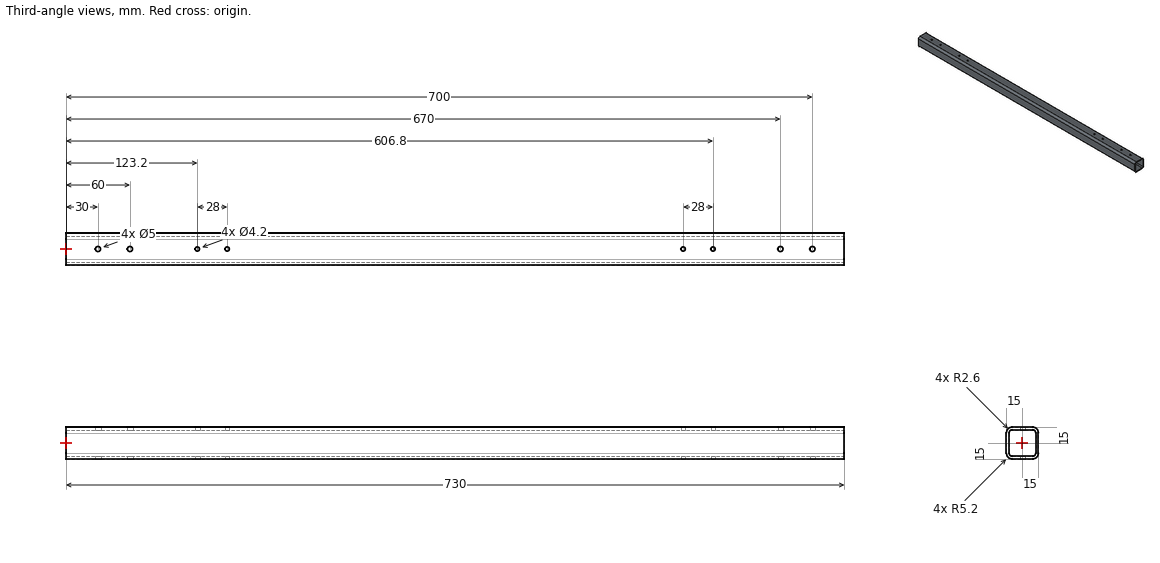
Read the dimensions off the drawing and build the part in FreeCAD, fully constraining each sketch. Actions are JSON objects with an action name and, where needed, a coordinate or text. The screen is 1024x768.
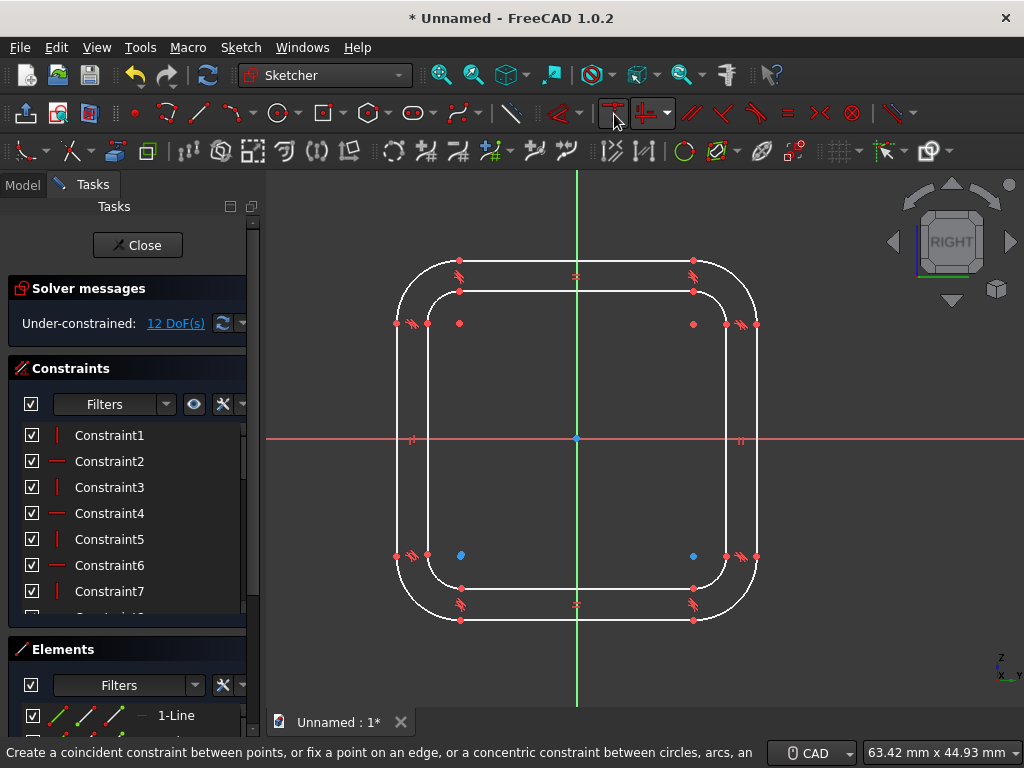
{"action": "left_click", "coordinate": [722, 613]}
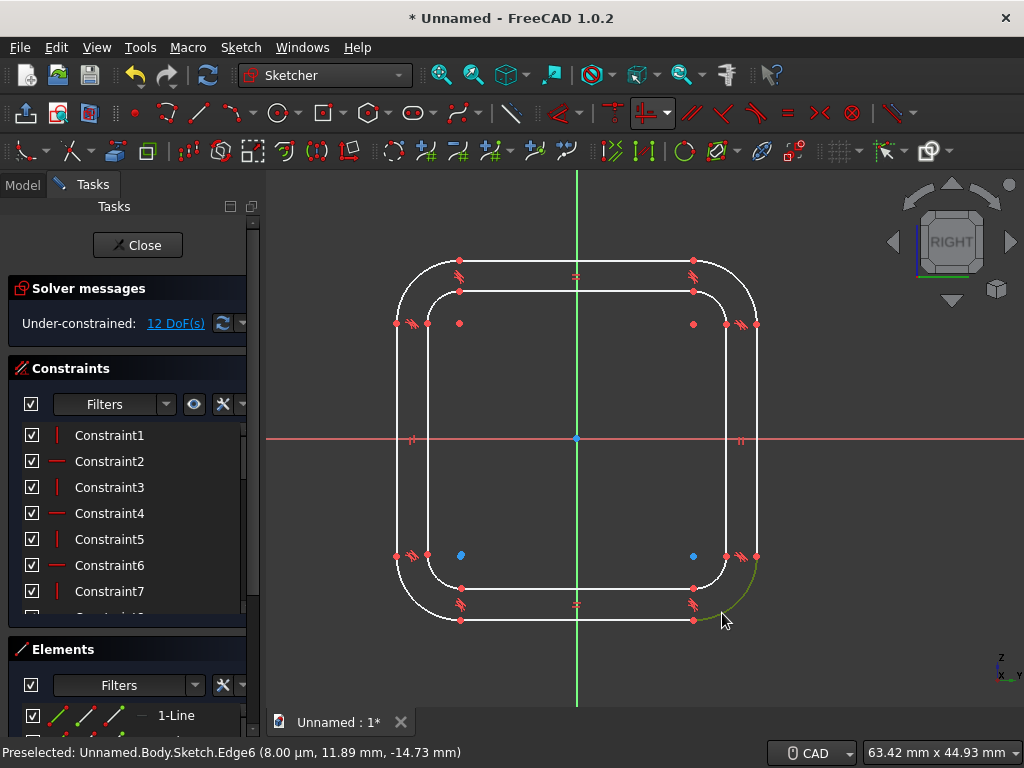
{"action": "left_click", "coordinate": [709, 585]}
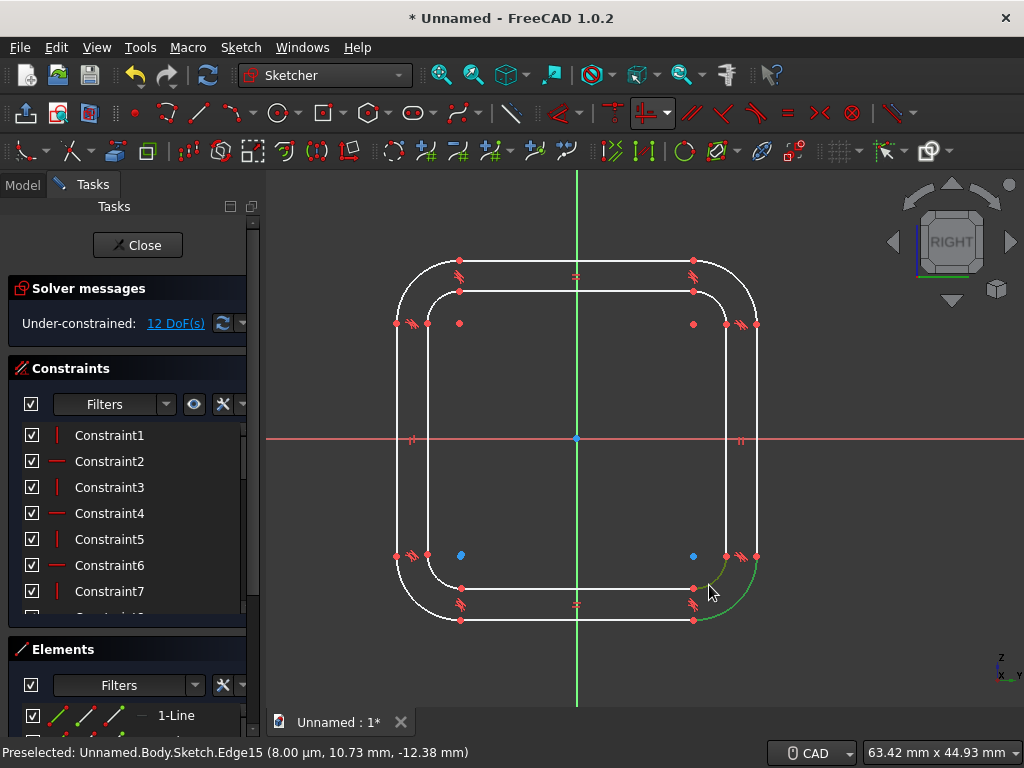
{"action": "left_click", "coordinate": [614, 114]}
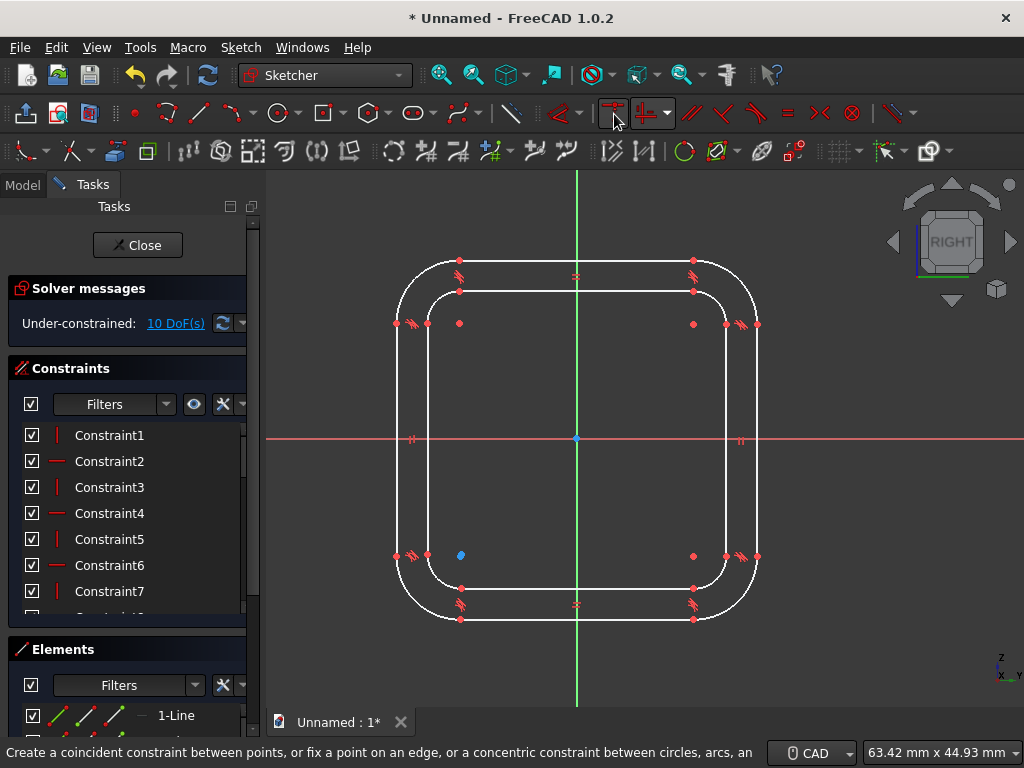
{"action": "left_click", "coordinate": [404, 585]}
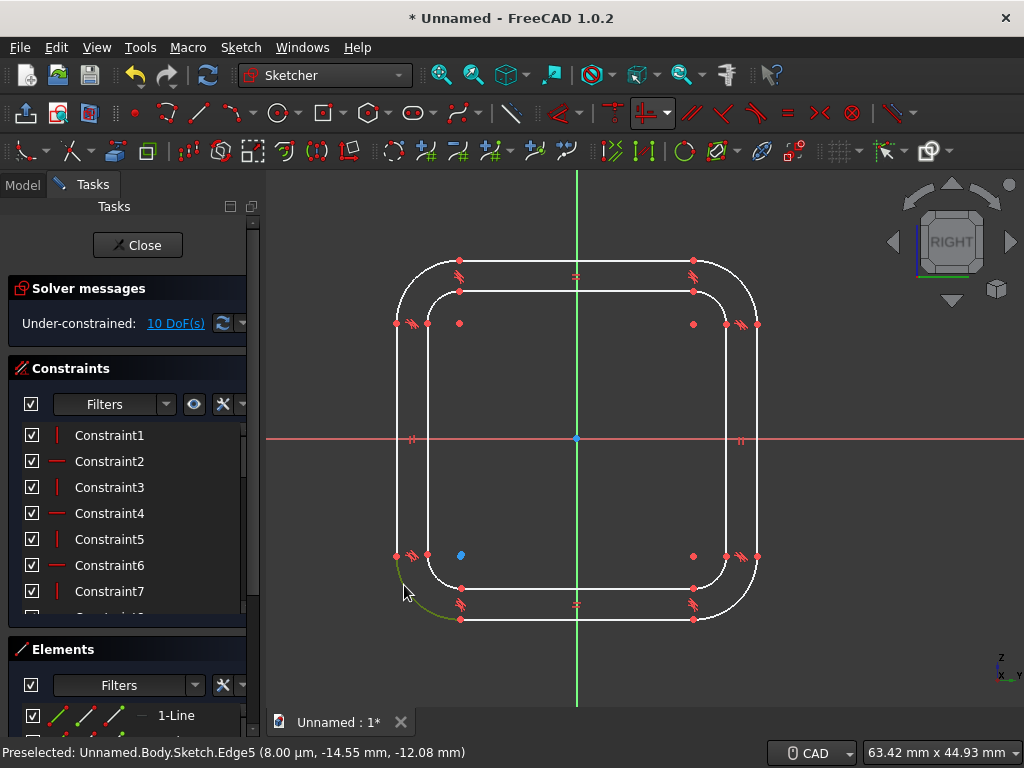
{"action": "left_click", "coordinate": [723, 613]}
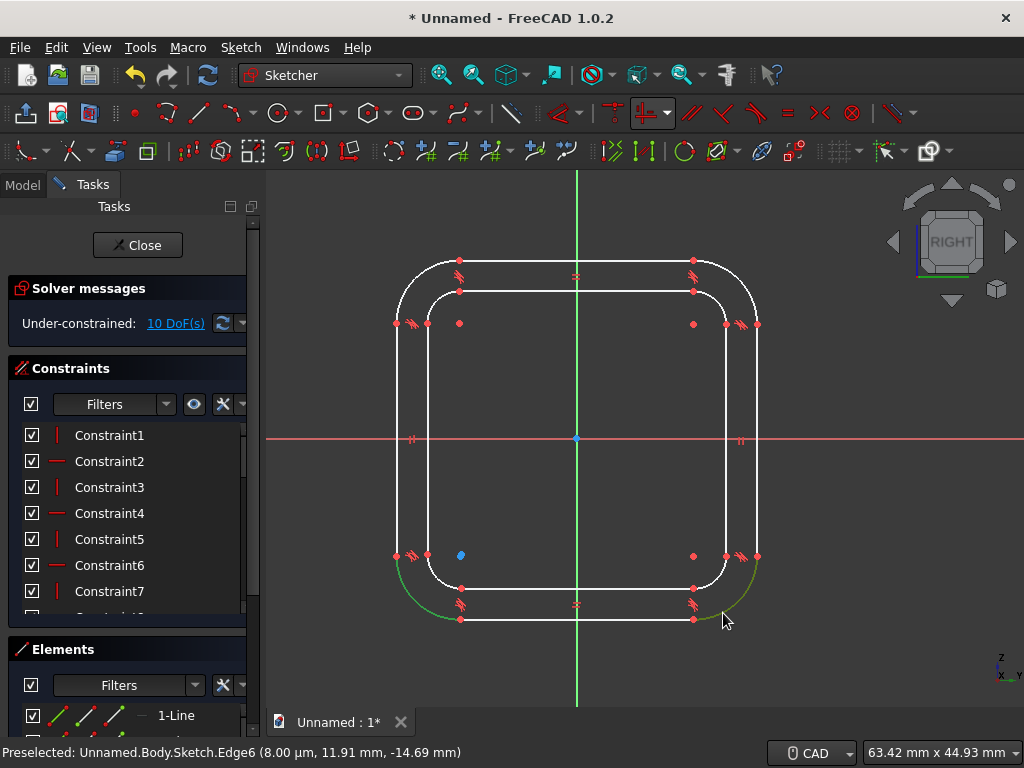
{"action": "left_click", "coordinate": [750, 295]}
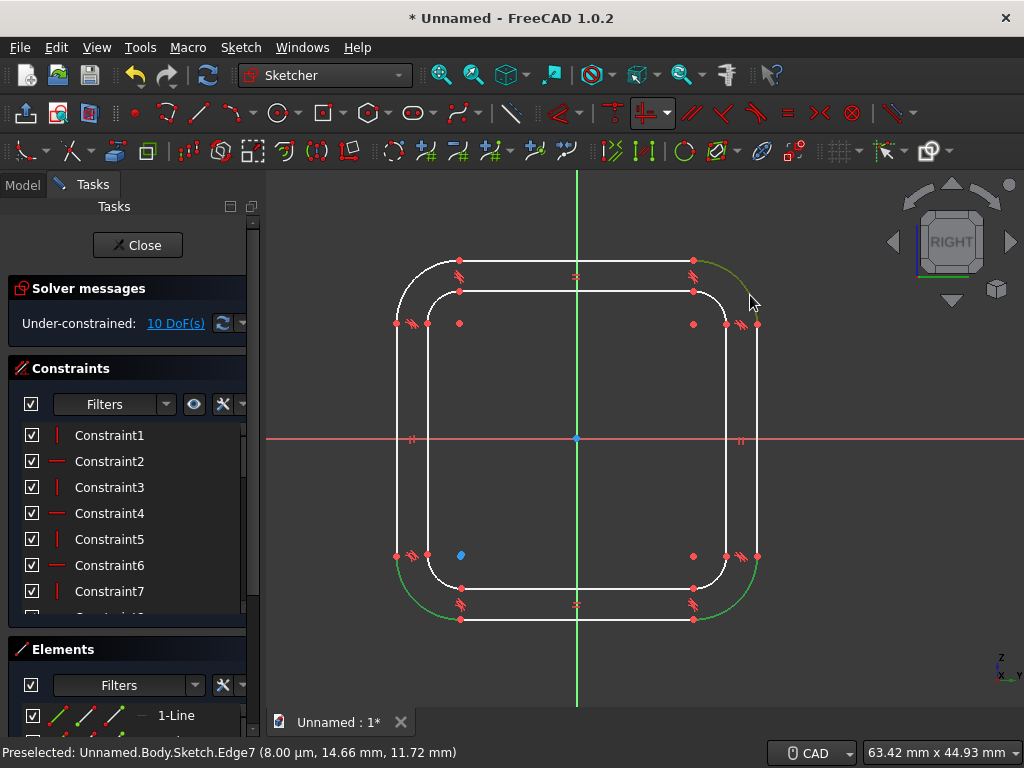
{"action": "left_click", "coordinate": [431, 267]}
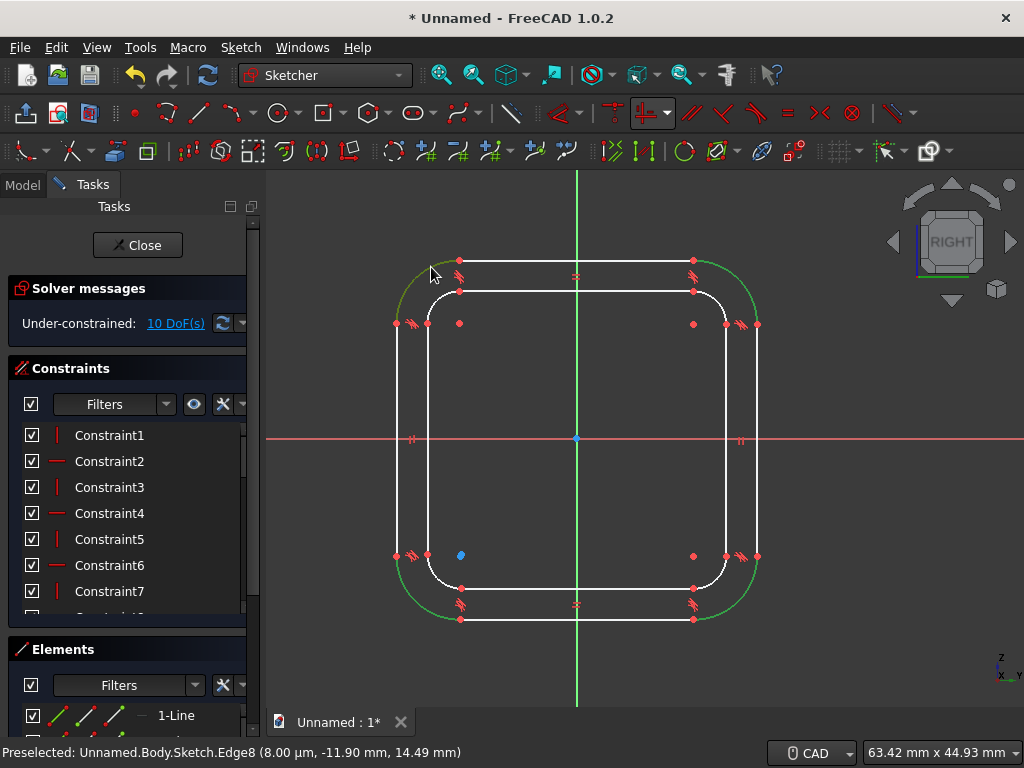
{"action": "left_click", "coordinate": [788, 114]}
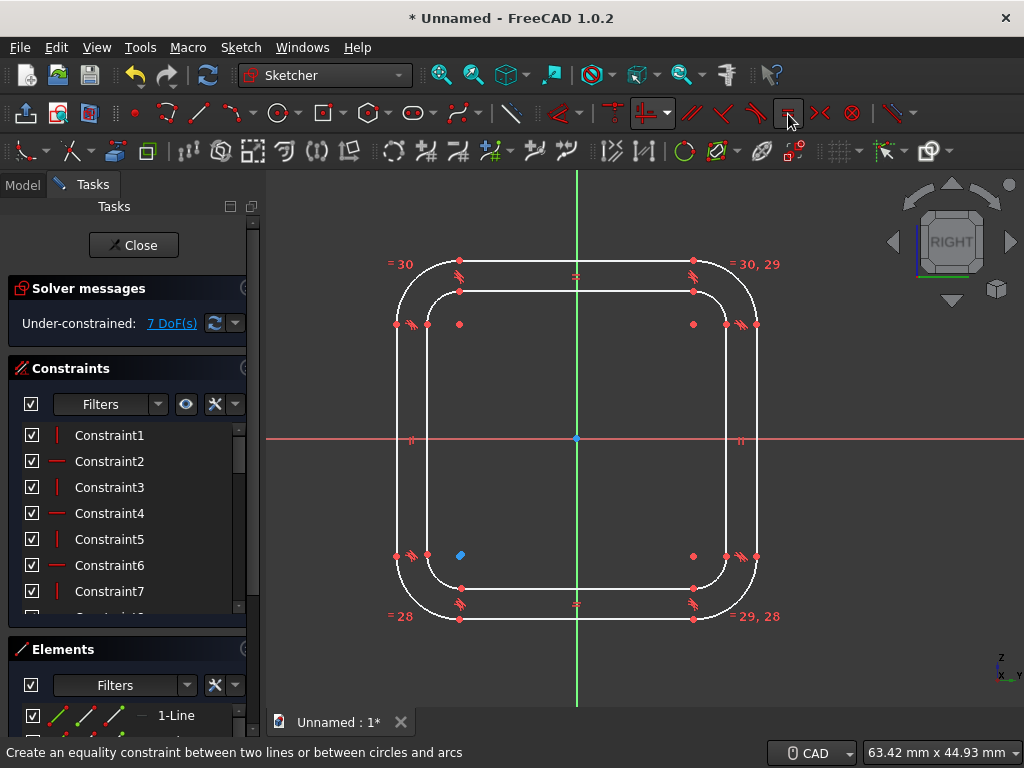
{"action": "left_click", "coordinate": [445, 295]}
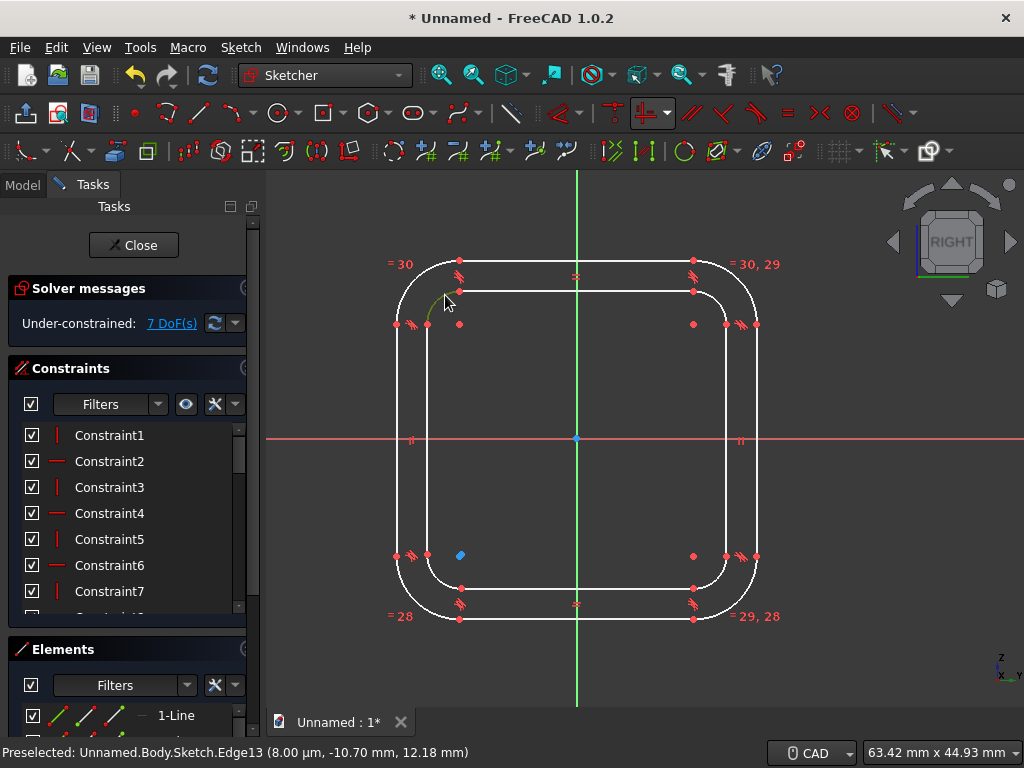
{"action": "left_click", "coordinate": [431, 570]}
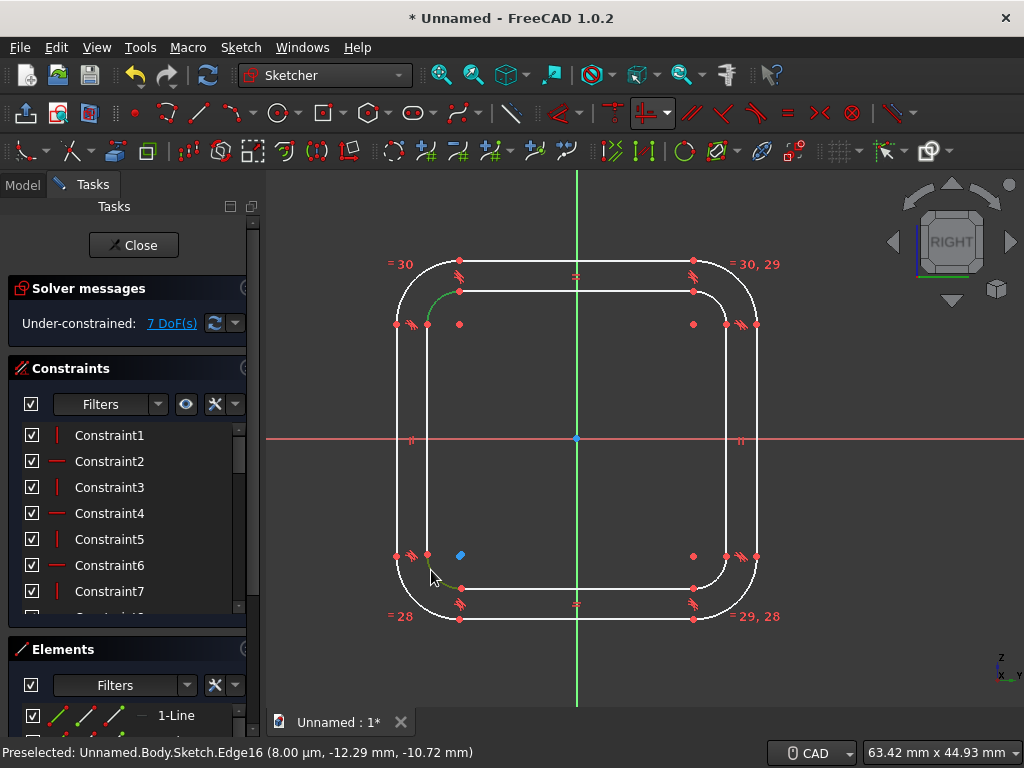
{"action": "left_click", "coordinate": [788, 114]}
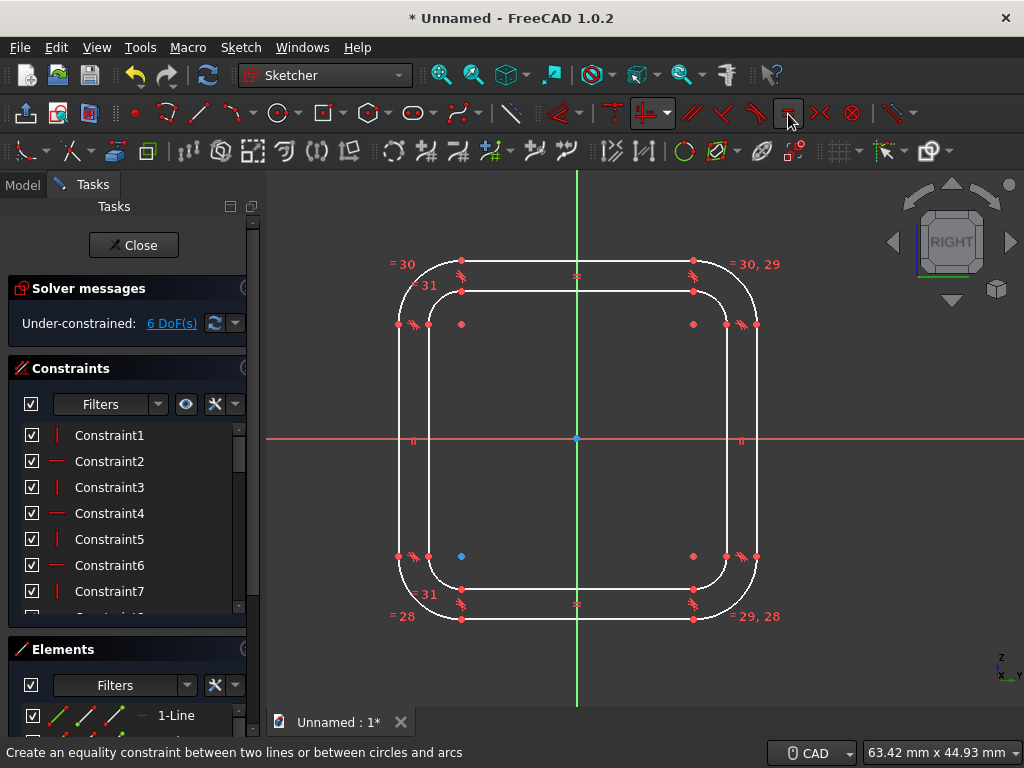
{"action": "left_click", "coordinate": [558, 114]}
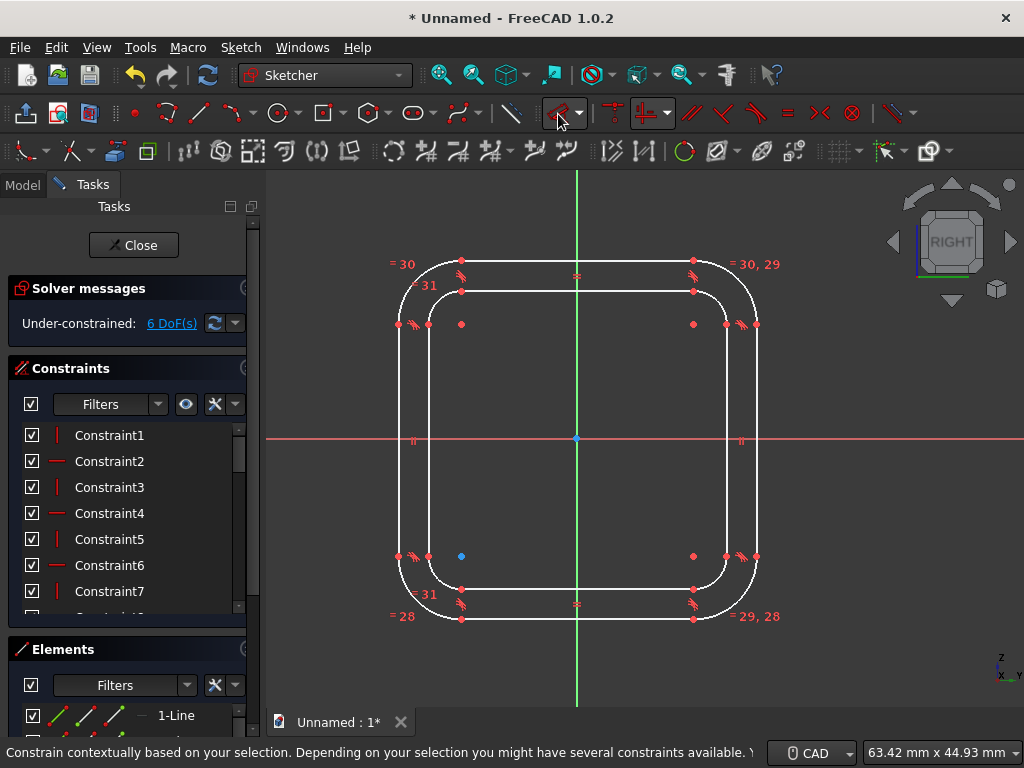
{"action": "left_click", "coordinate": [405, 585]}
{"action": "left_click", "coordinate": [376, 599]}